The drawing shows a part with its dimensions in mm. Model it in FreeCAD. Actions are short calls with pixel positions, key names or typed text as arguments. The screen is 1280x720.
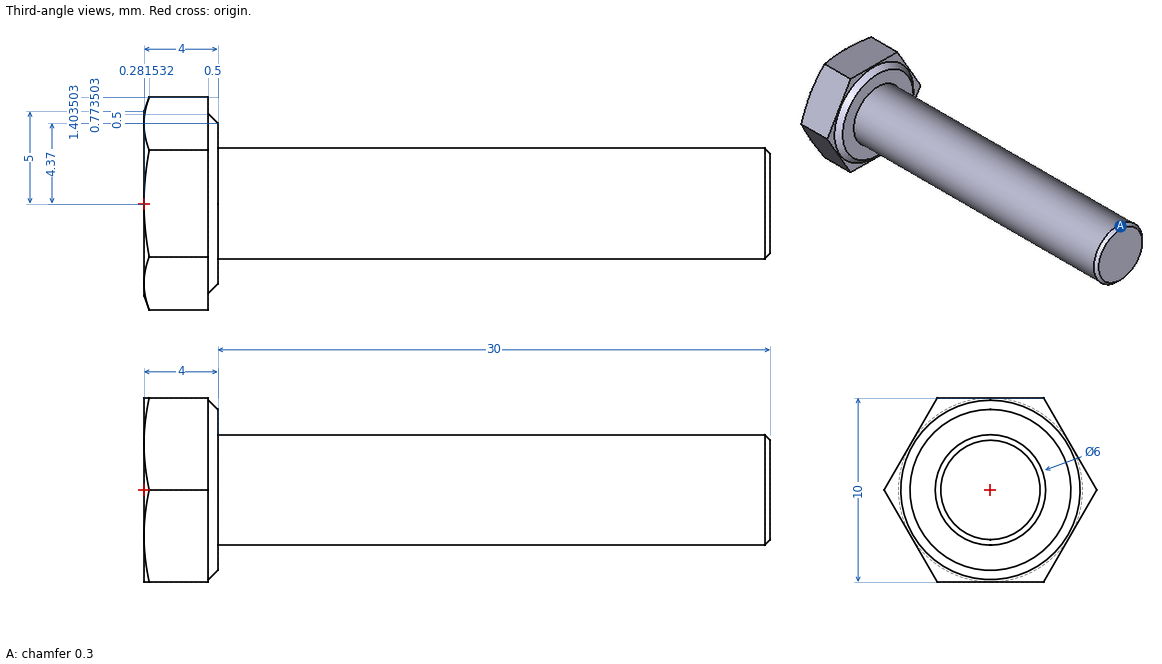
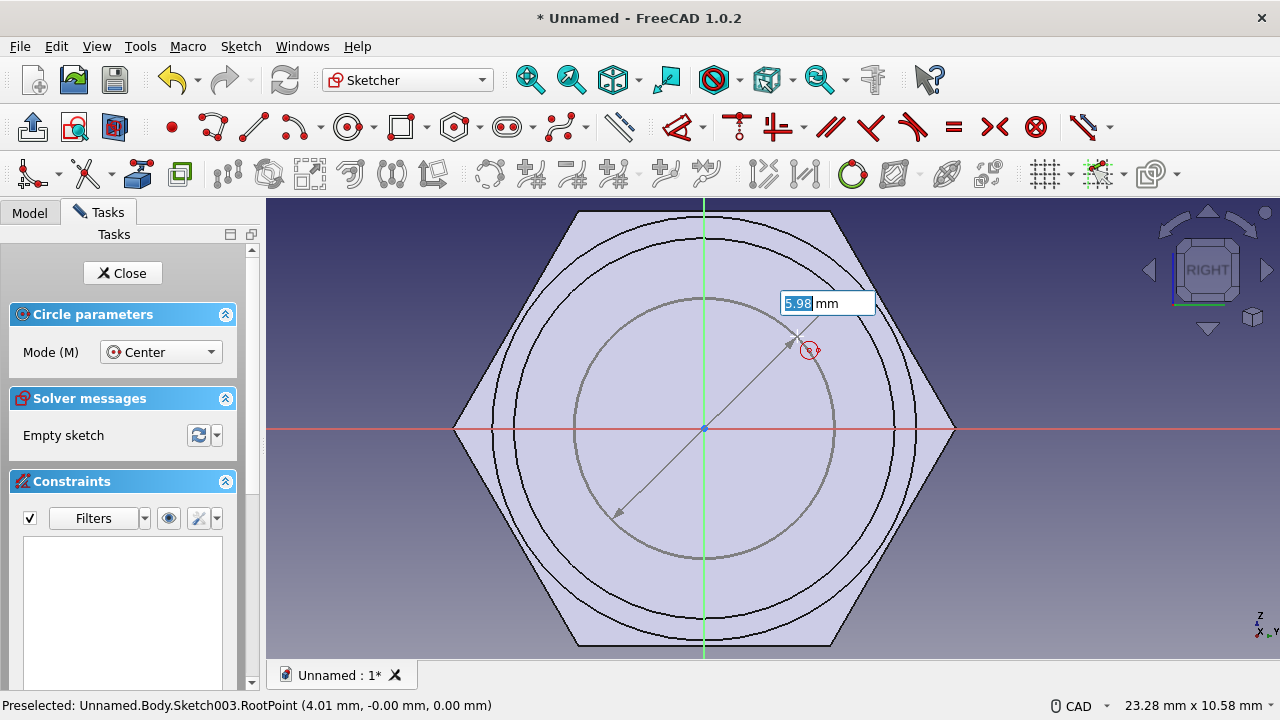
text(6)
key(Return)
key(Escape)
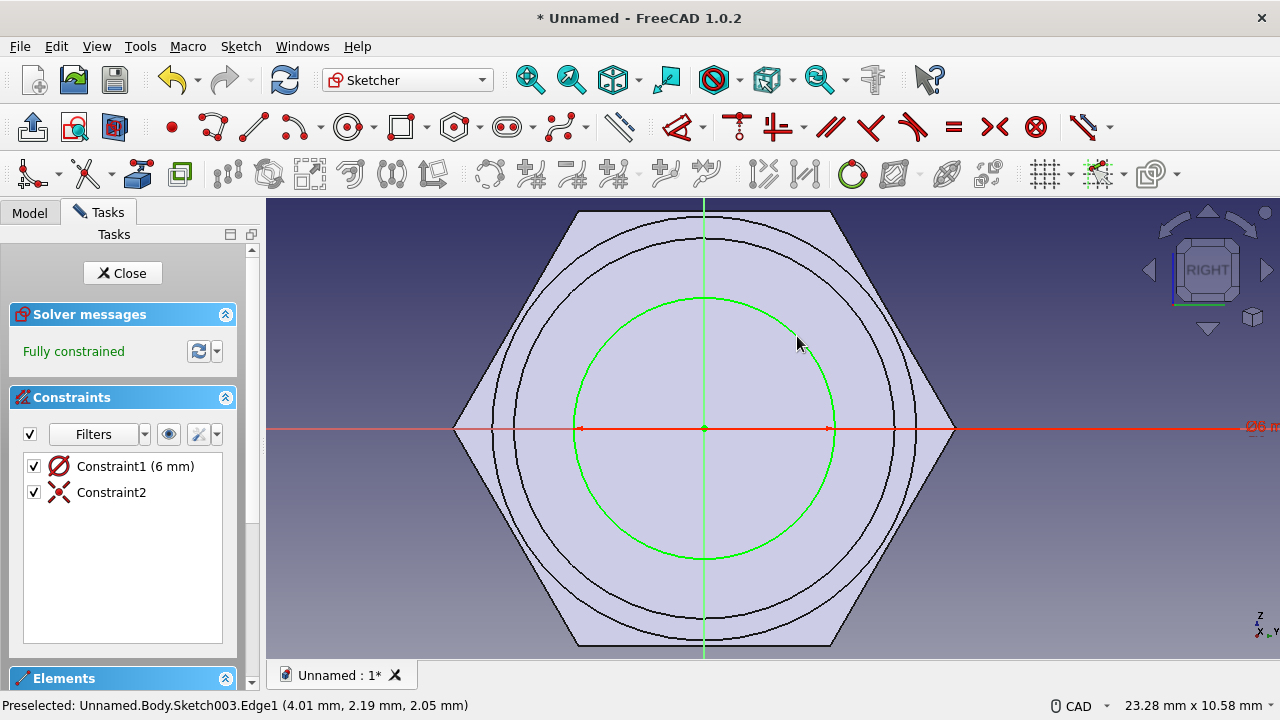
click(123, 273)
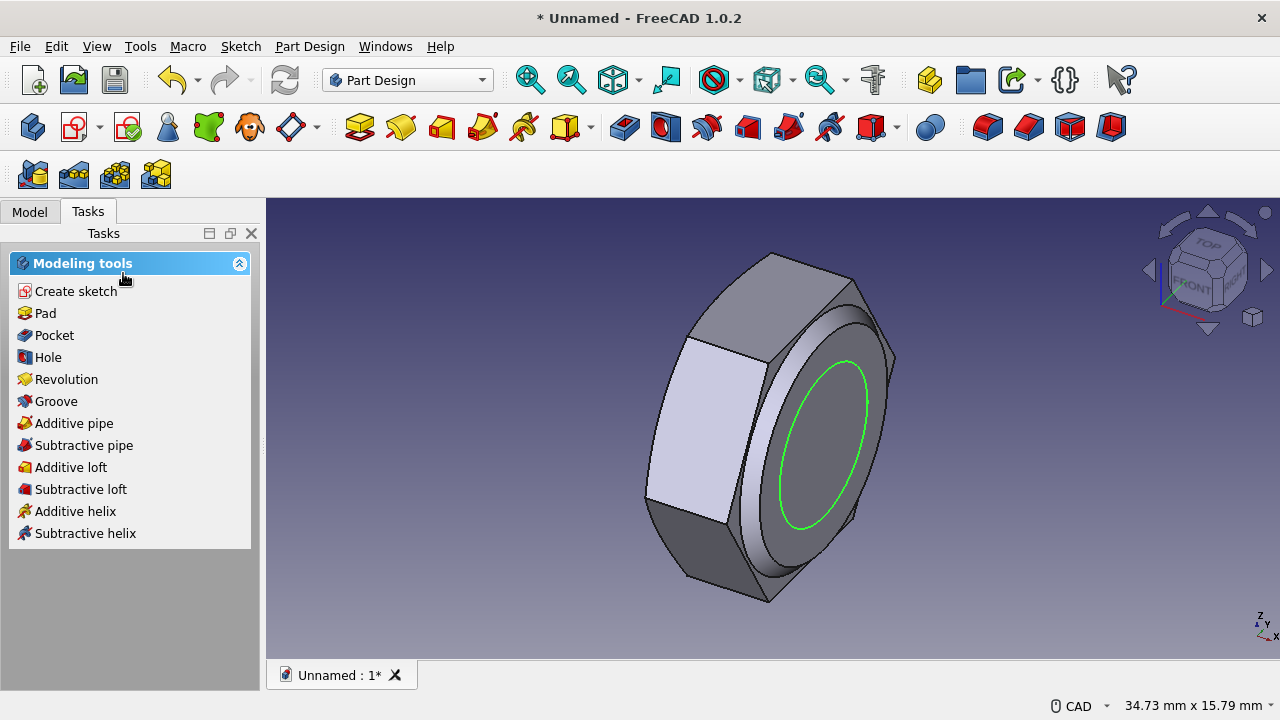
click(360, 128)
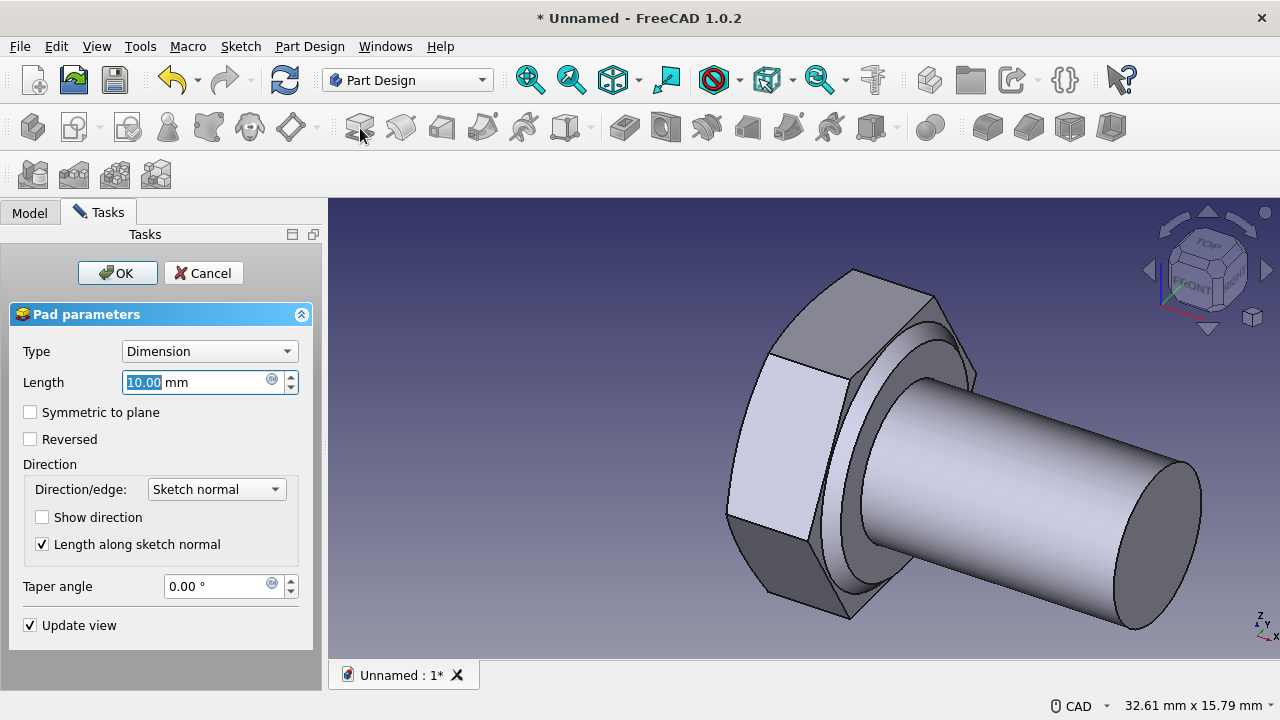
text(30)
key(Tab)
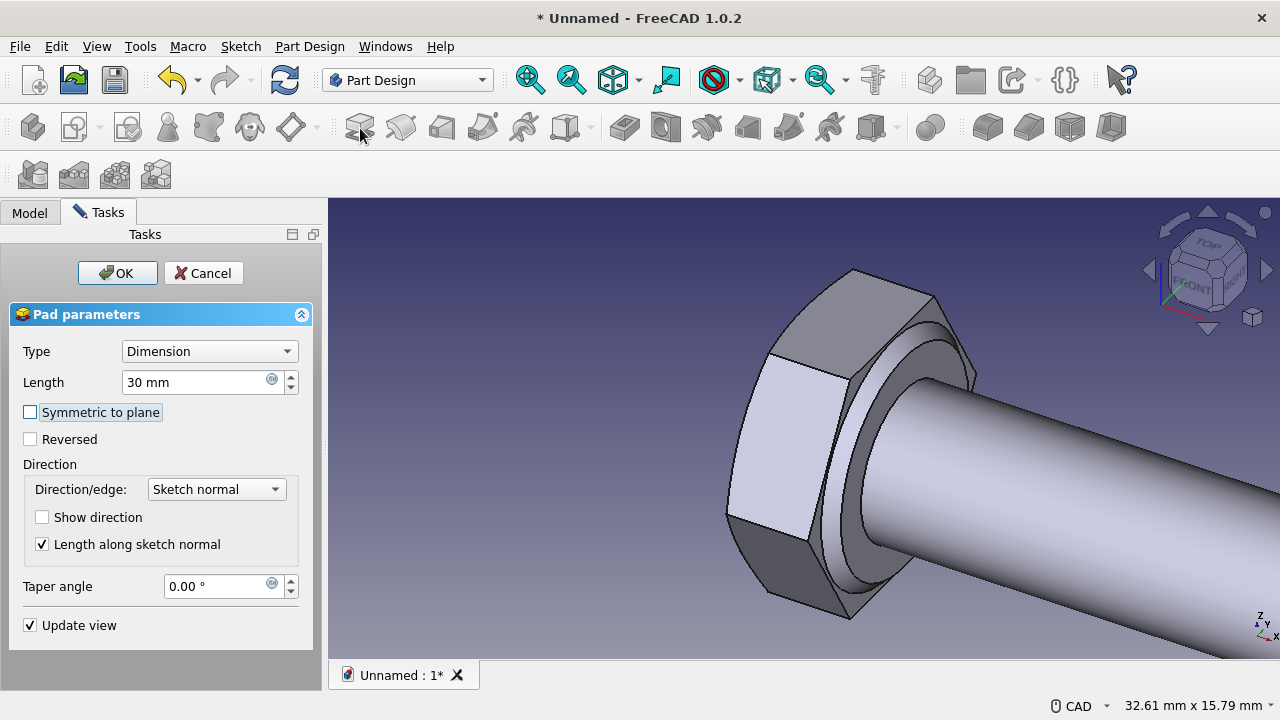
click(118, 273)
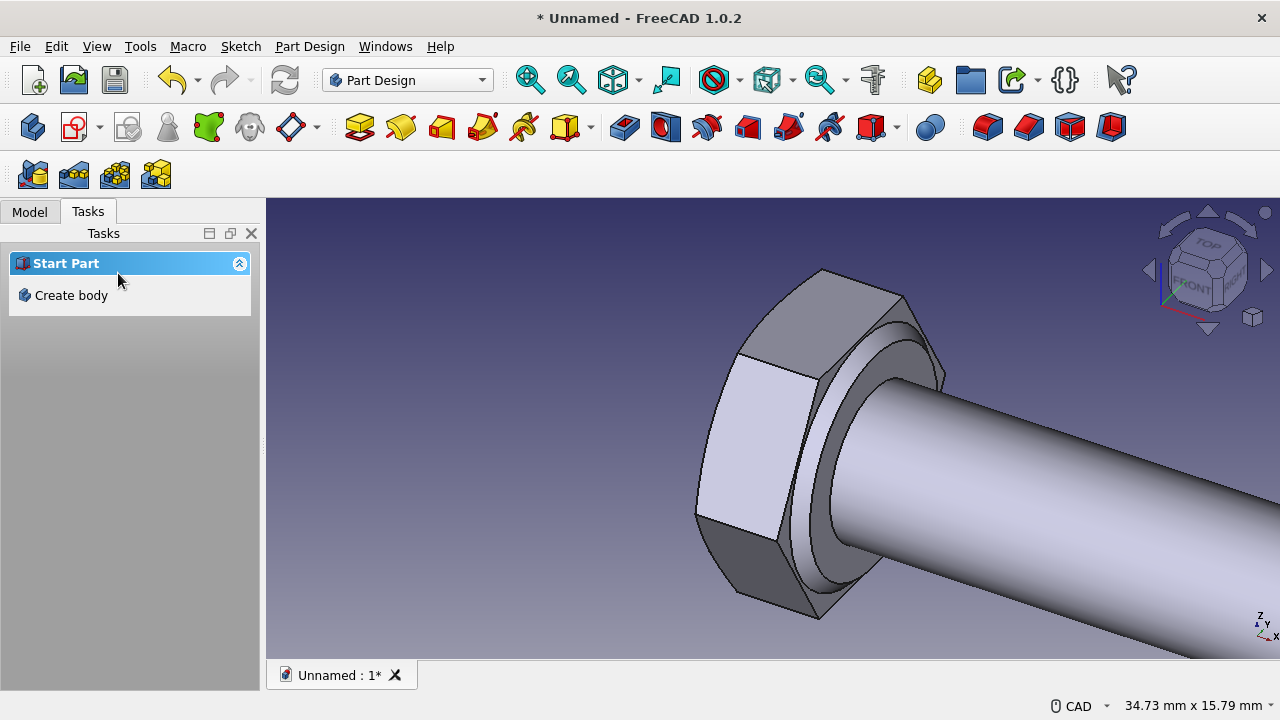
click(531, 80)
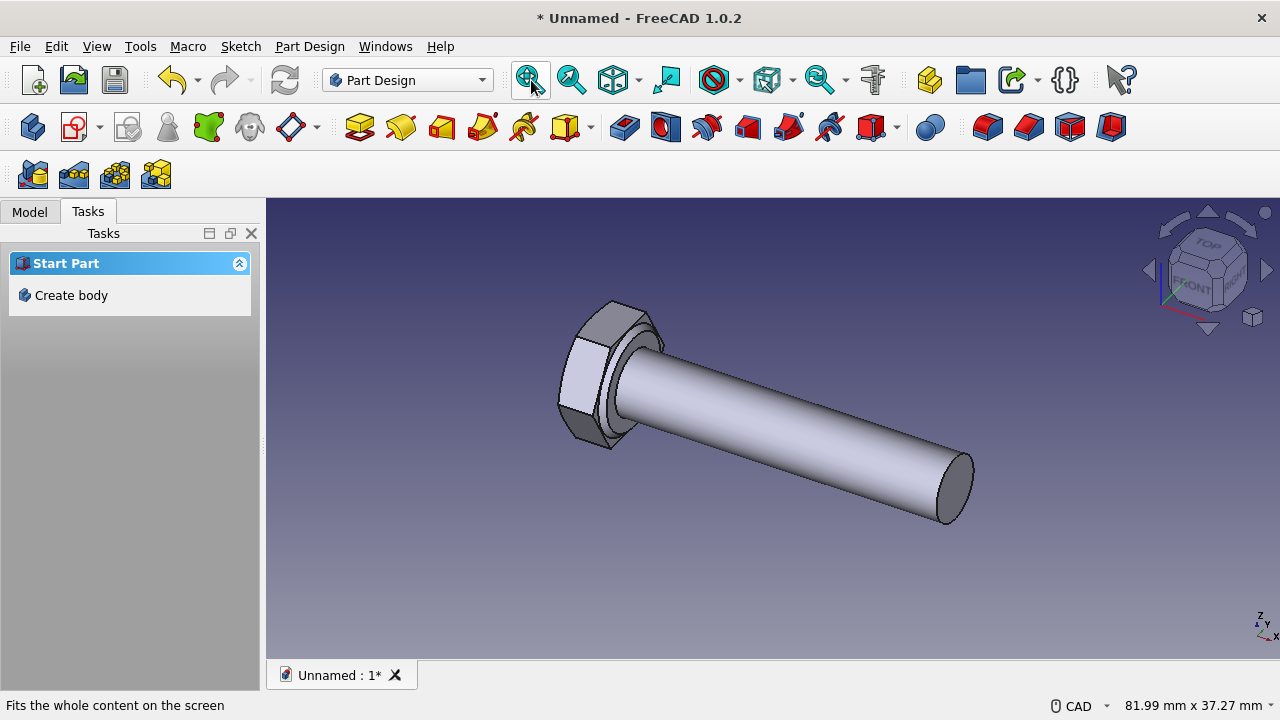
click(937, 506)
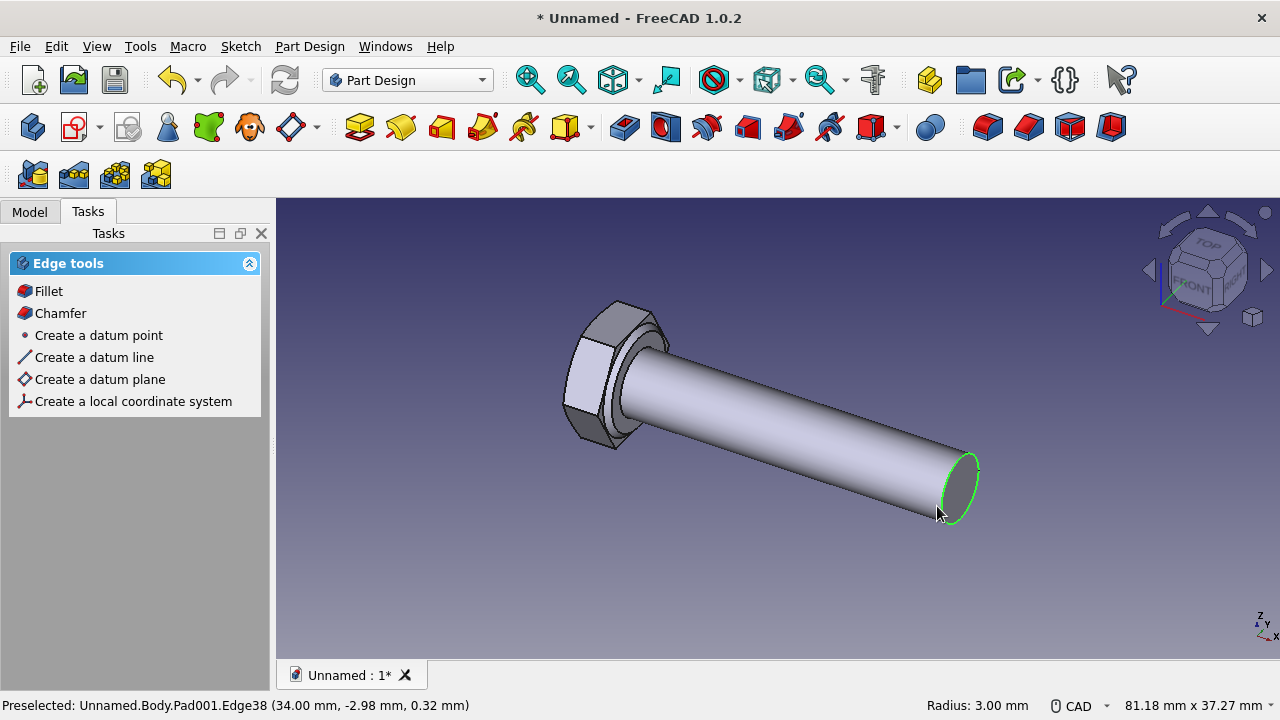
click(1029, 128)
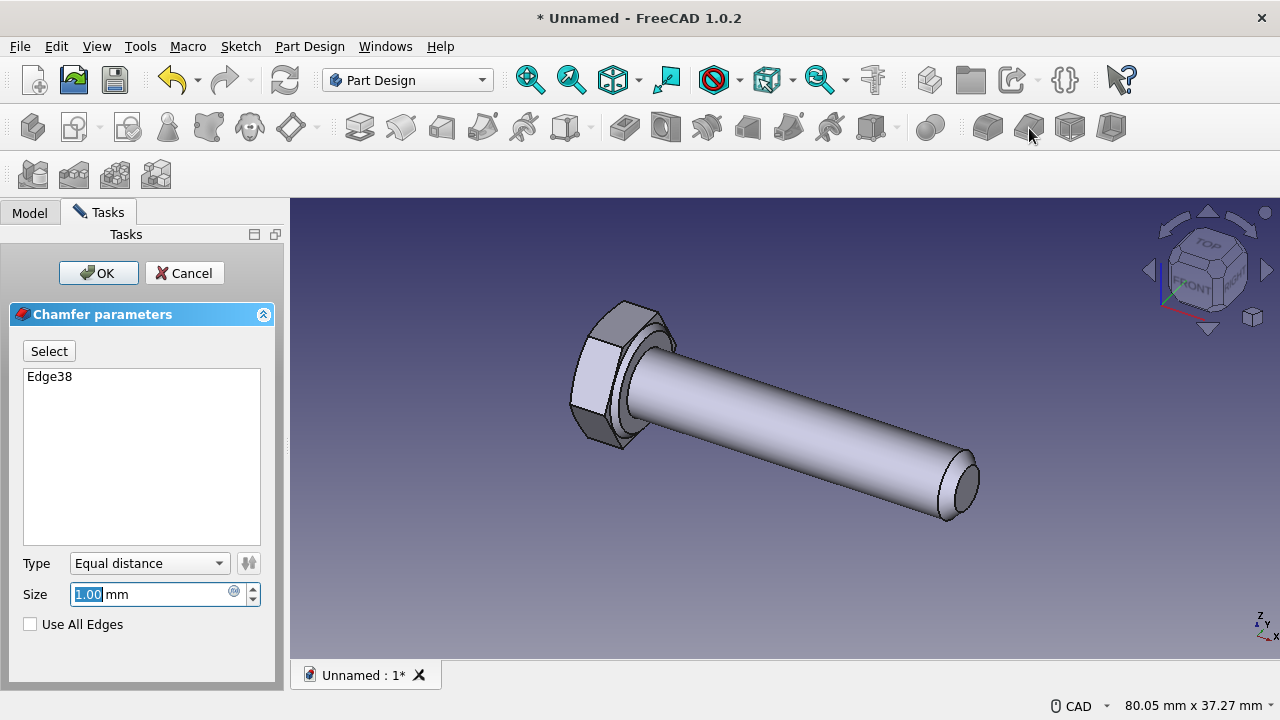
text(0.3)
key(Tab)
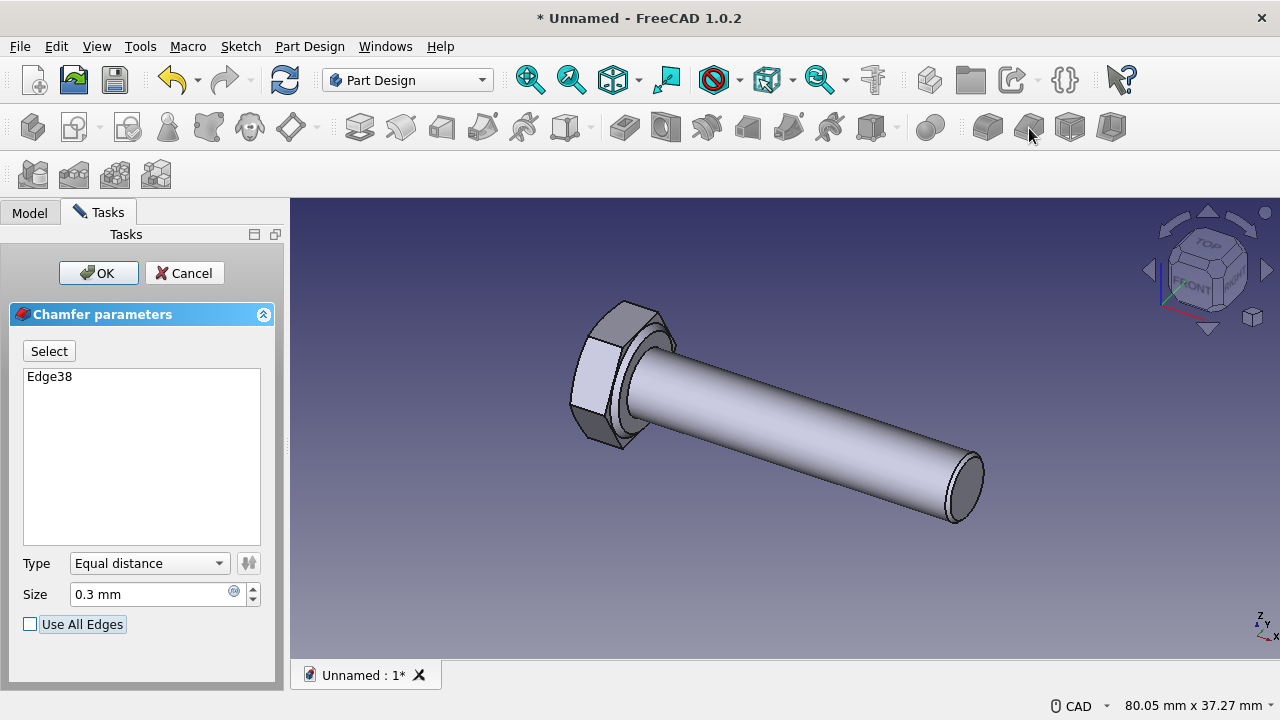
click(99, 273)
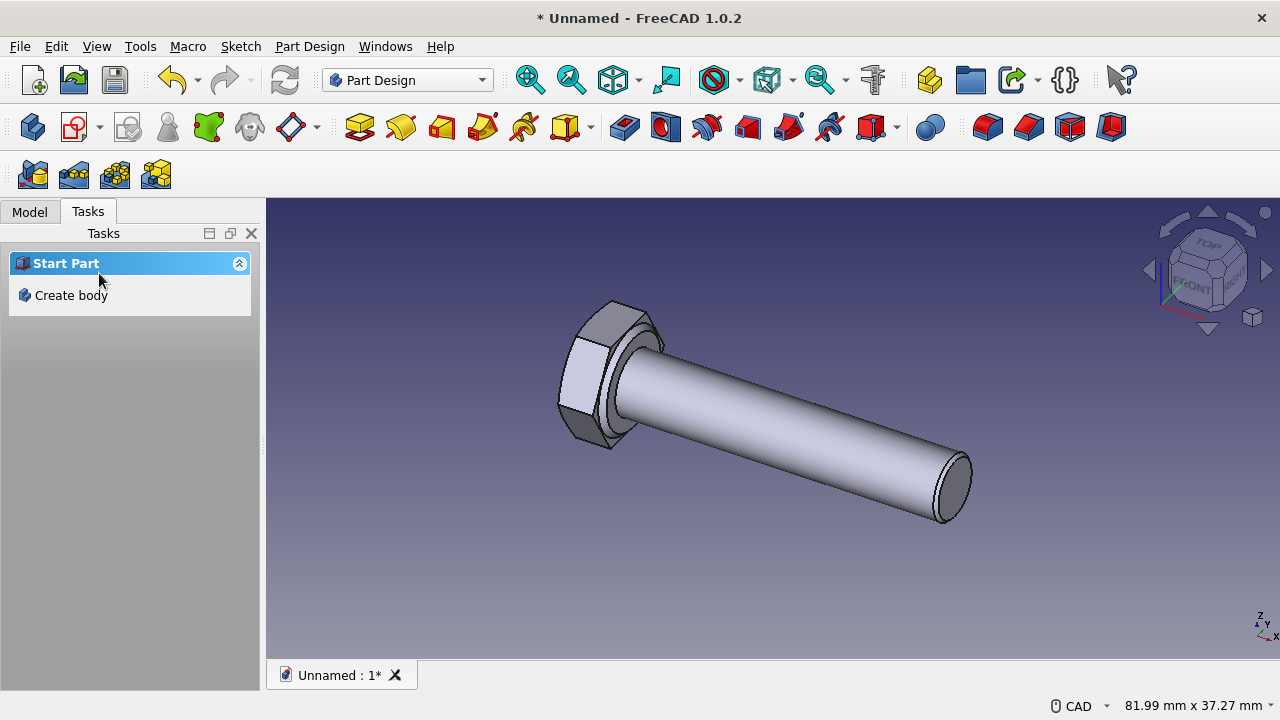
key(0)